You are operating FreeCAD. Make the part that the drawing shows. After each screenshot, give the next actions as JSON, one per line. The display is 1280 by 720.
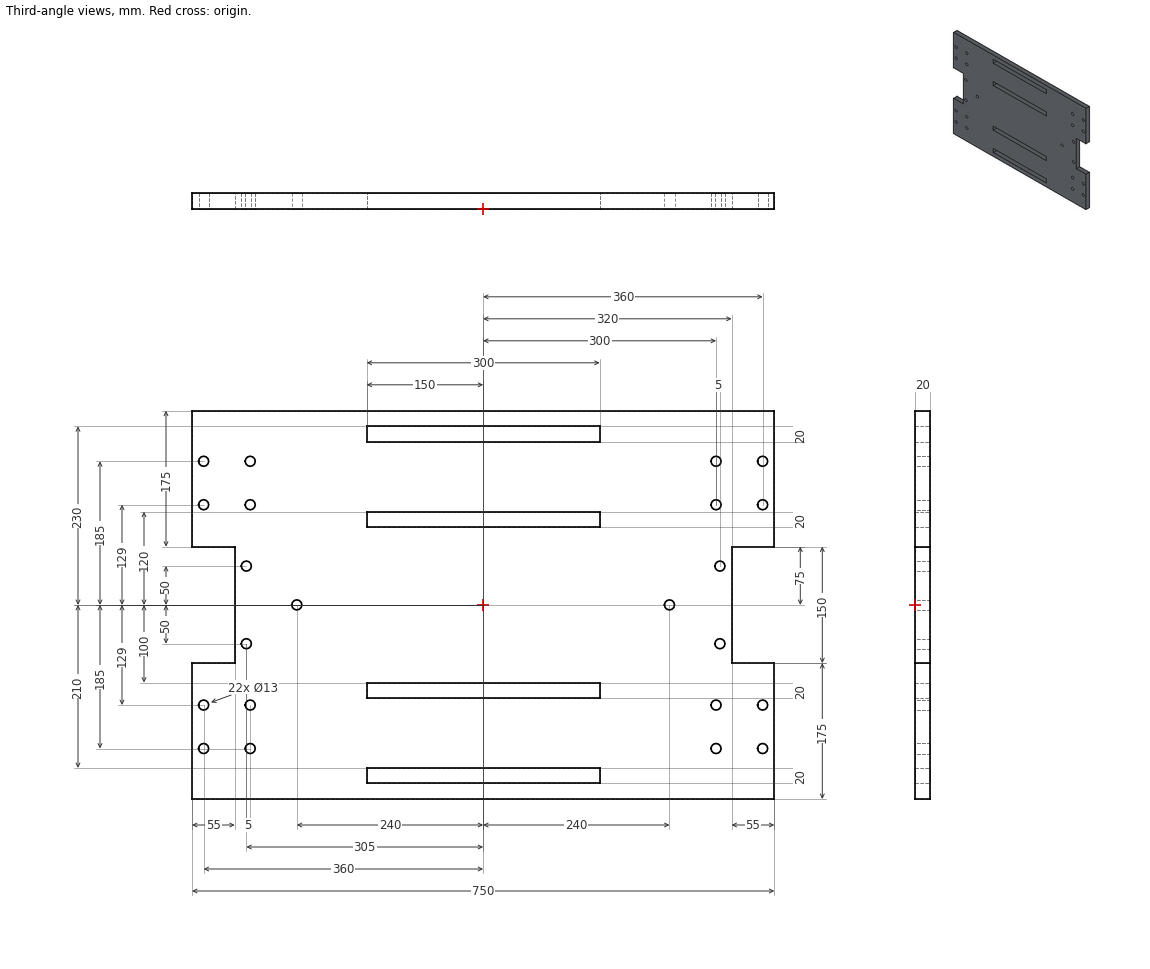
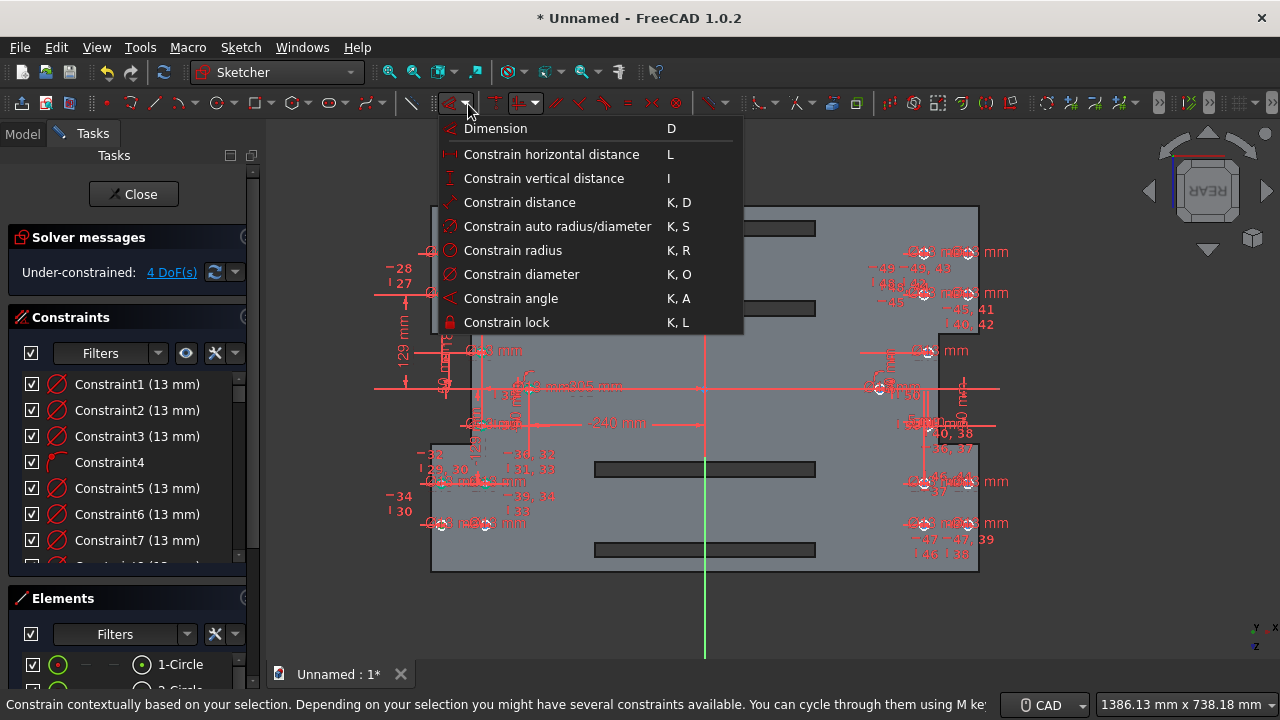
{"action": "left_click", "coordinate": [591, 178]}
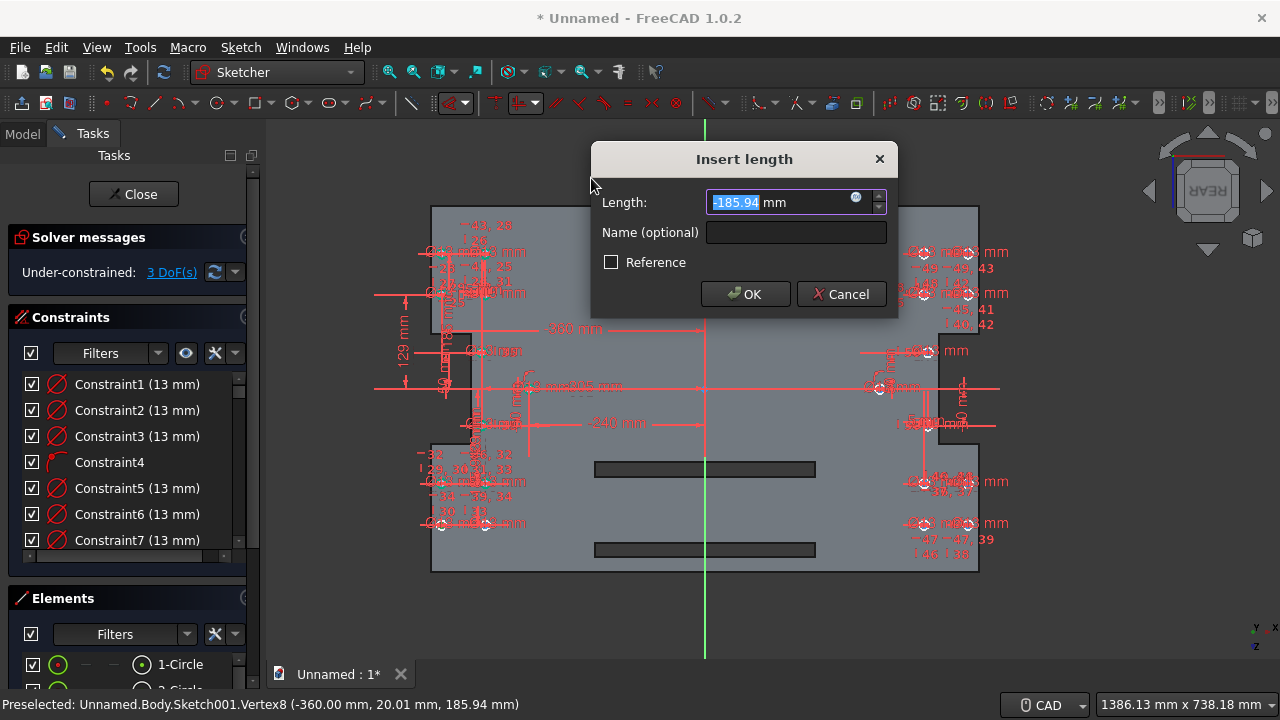
{"action": "type", "text": "-185"}
{"action": "key", "text": "Return"}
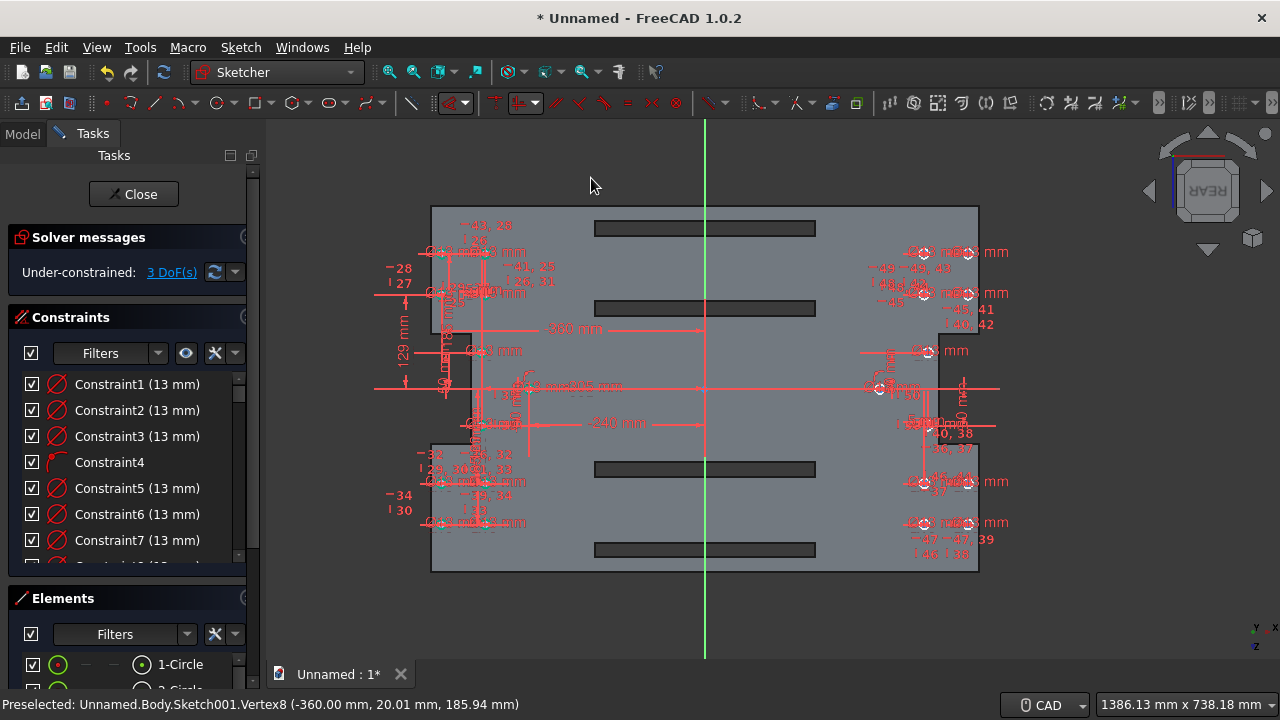
{"action": "left_click", "coordinate": [968, 484]}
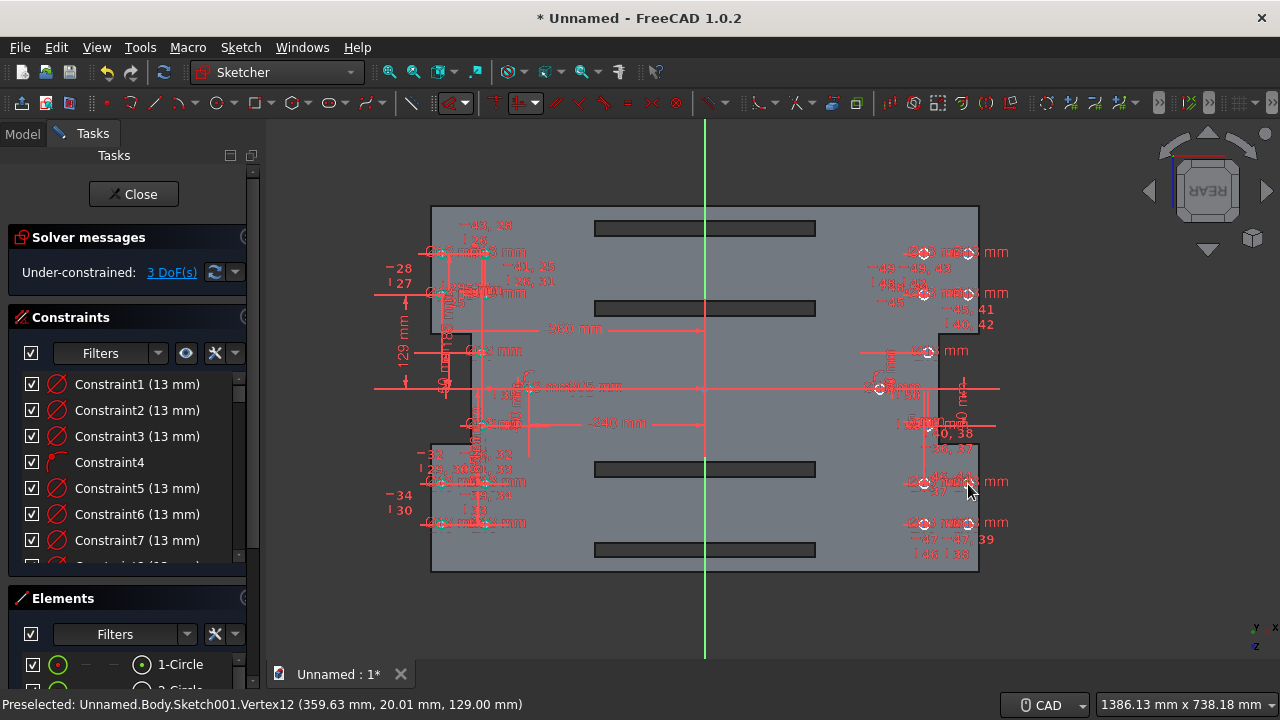
{"action": "left_click", "coordinate": [468, 104]}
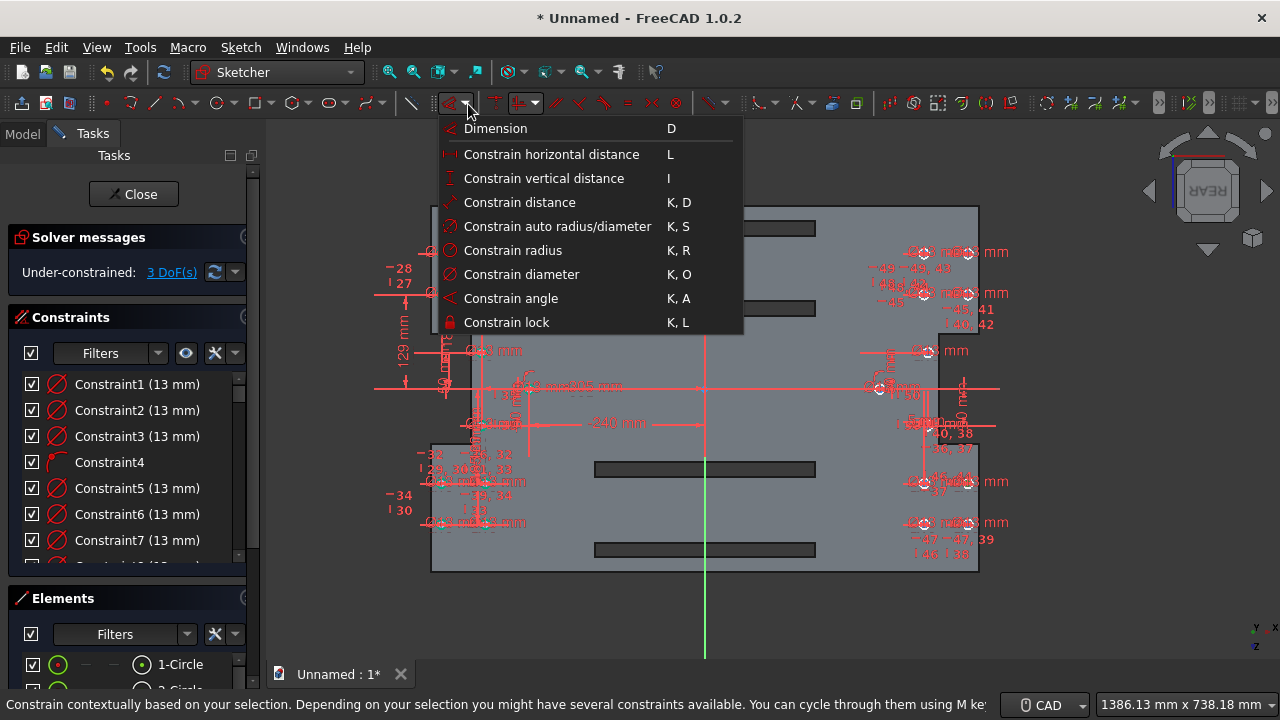
{"action": "left_click", "coordinate": [591, 154]}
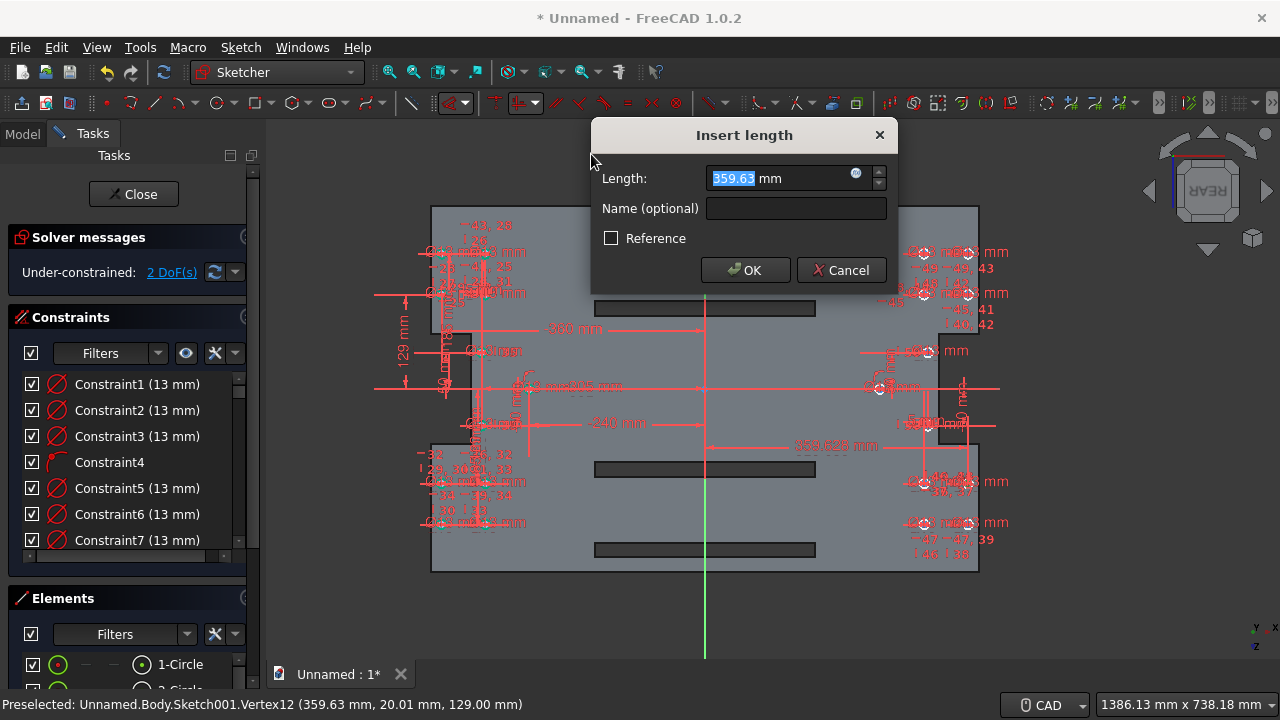
{"action": "type", "text": "360"}
{"action": "key", "text": "Return"}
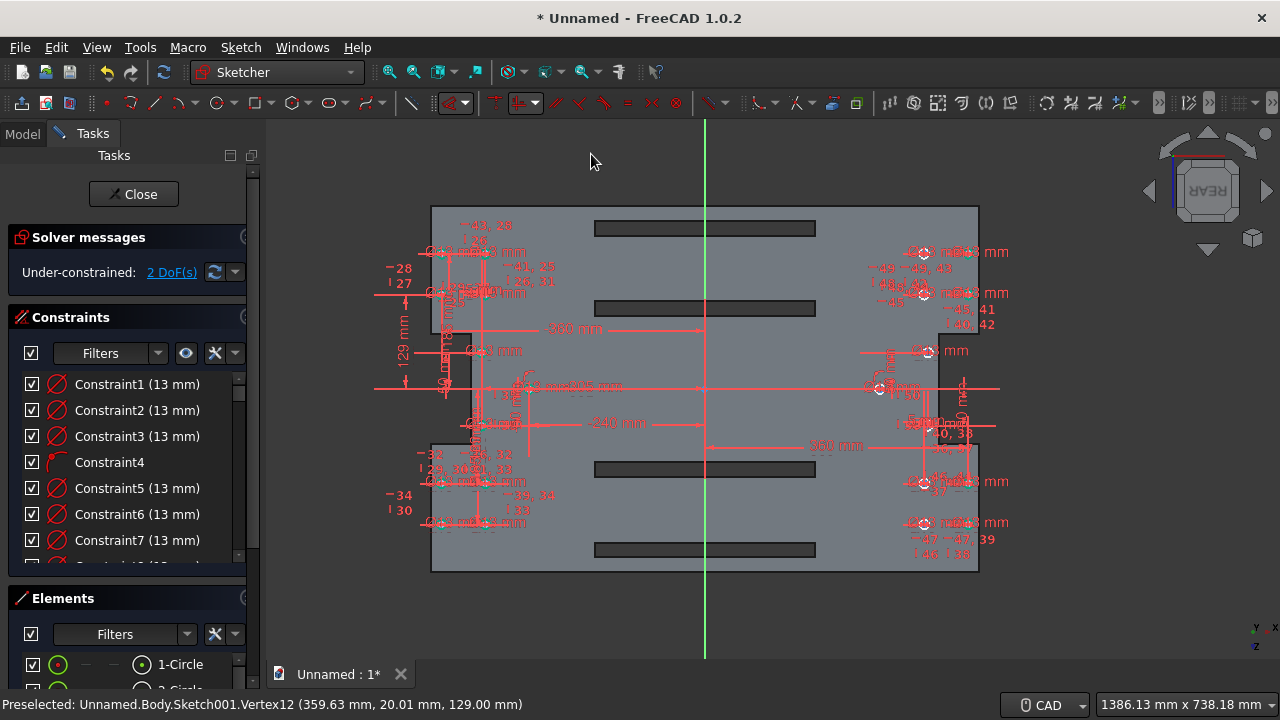
{"action": "left_click", "coordinate": [924, 484]}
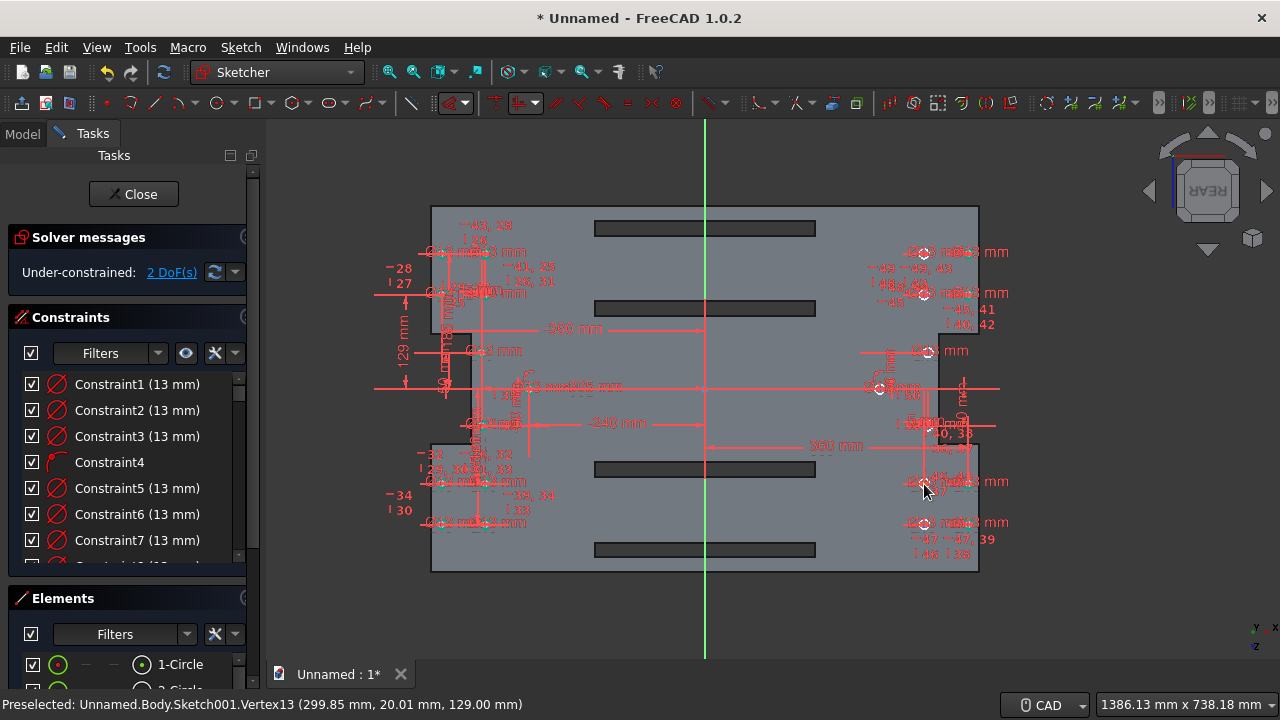
{"action": "key", "text": "l"}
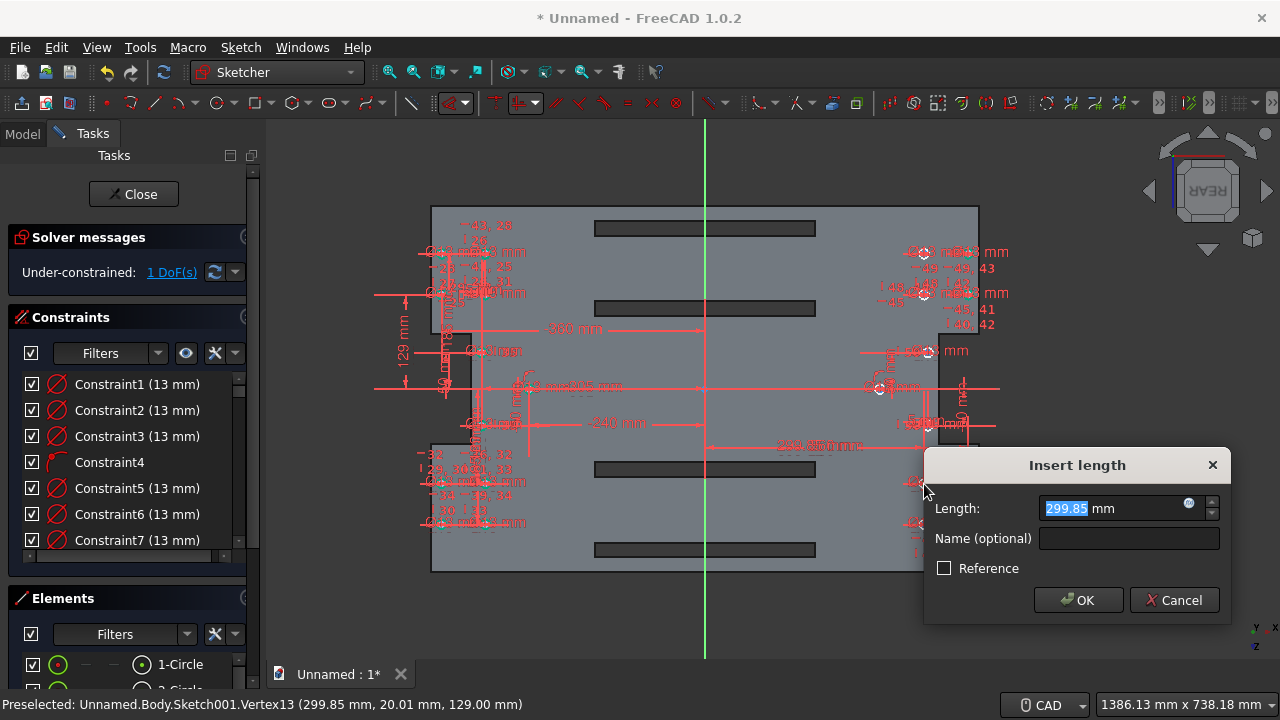
{"action": "type", "text": "300"}
{"action": "key", "text": "Return"}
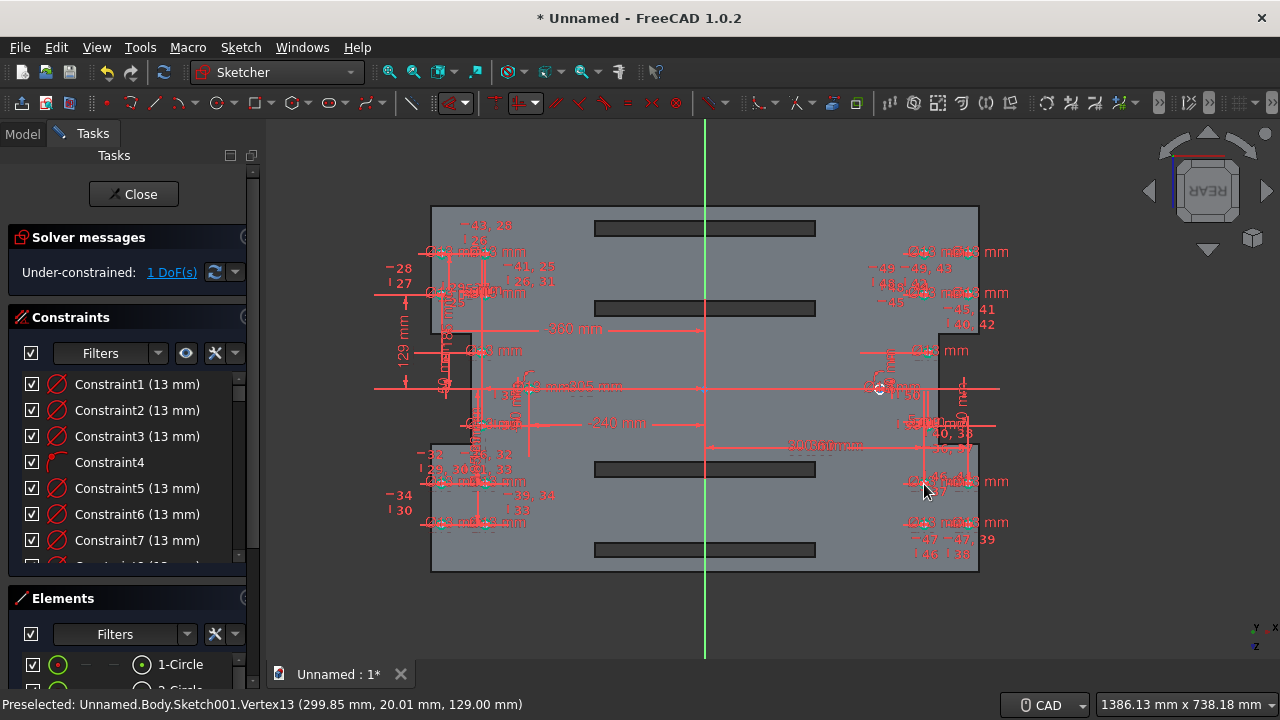
{"action": "left_click", "coordinate": [880, 389]}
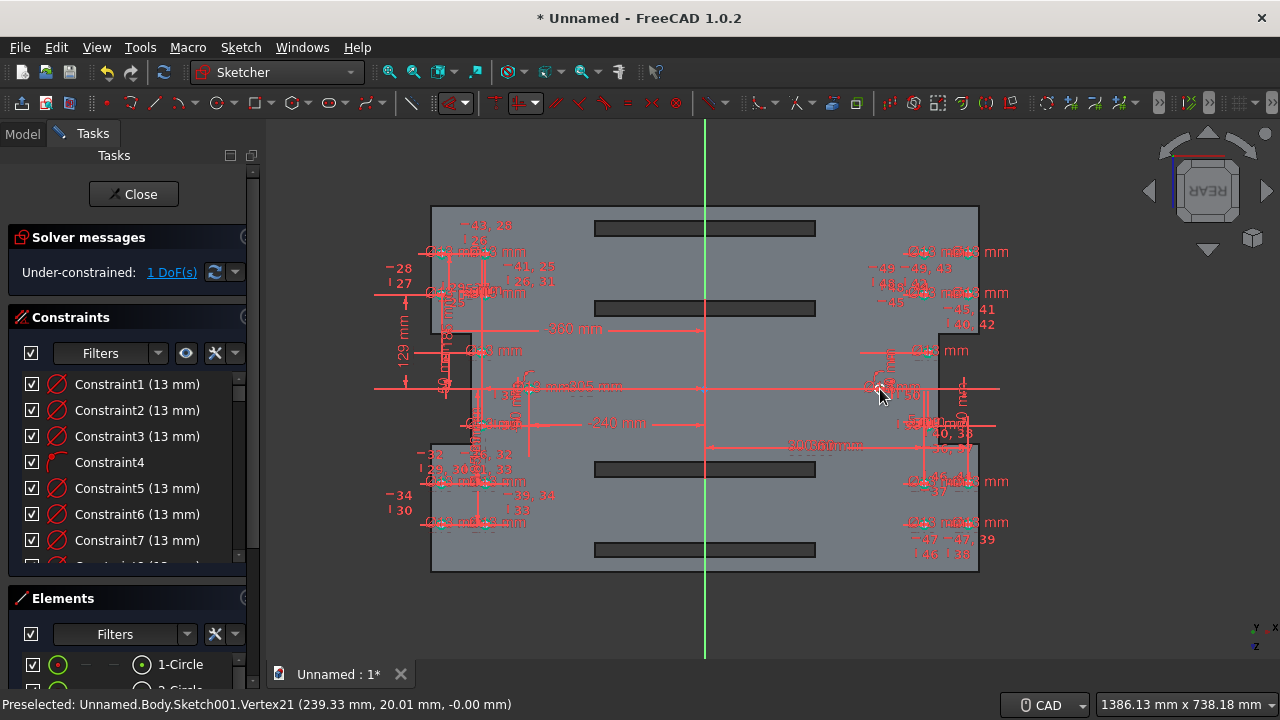
{"action": "left_click", "coordinate": [468, 104]}